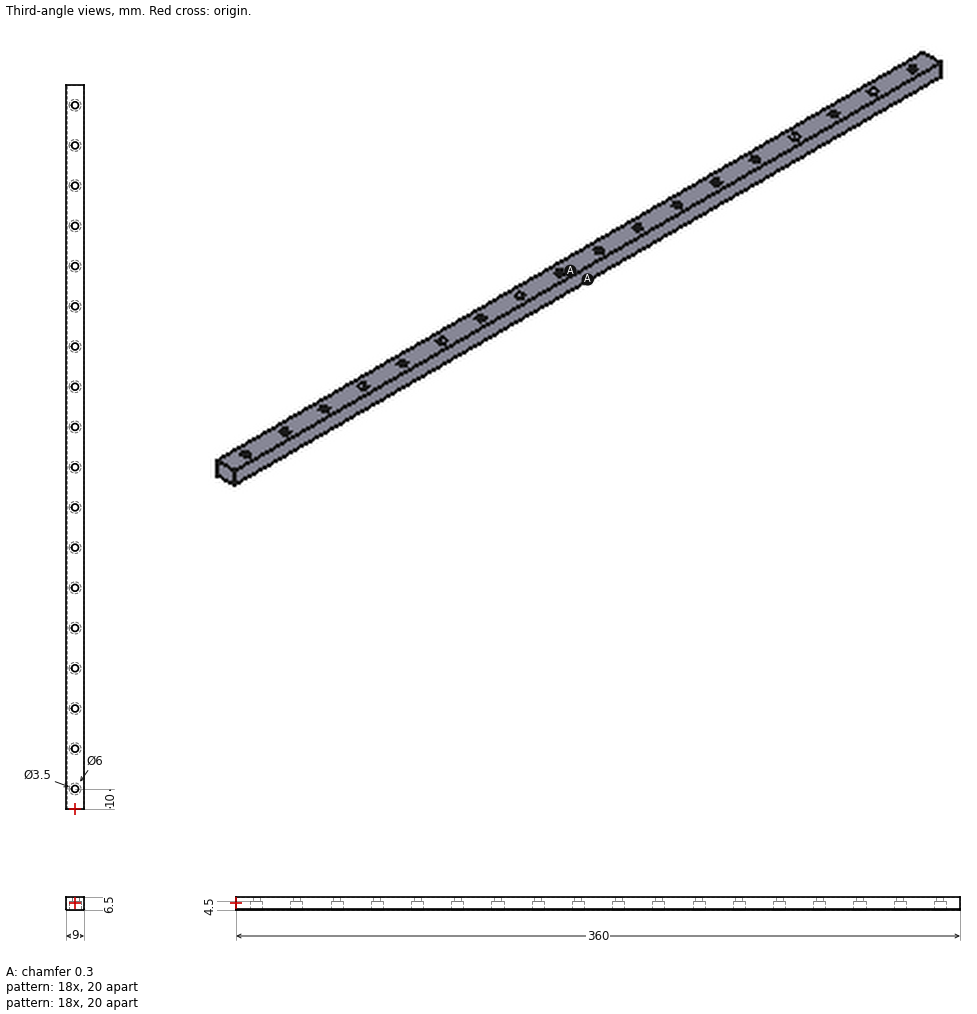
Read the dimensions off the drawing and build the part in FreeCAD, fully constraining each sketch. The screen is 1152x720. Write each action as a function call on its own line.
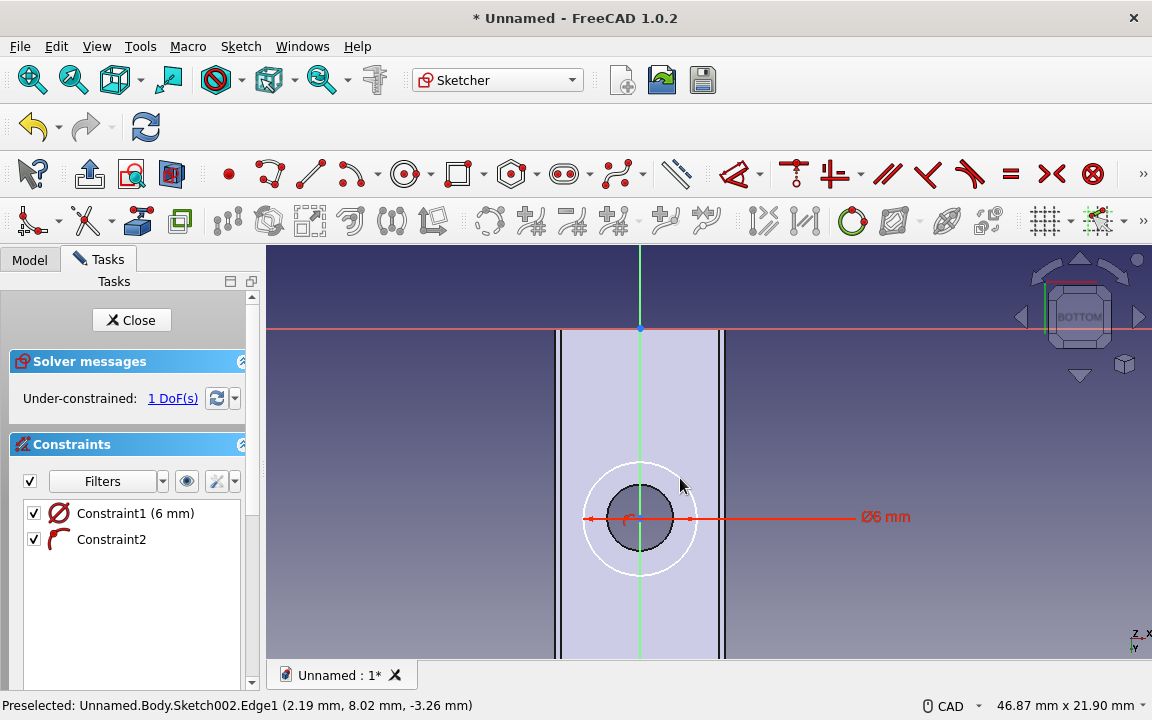
key(d)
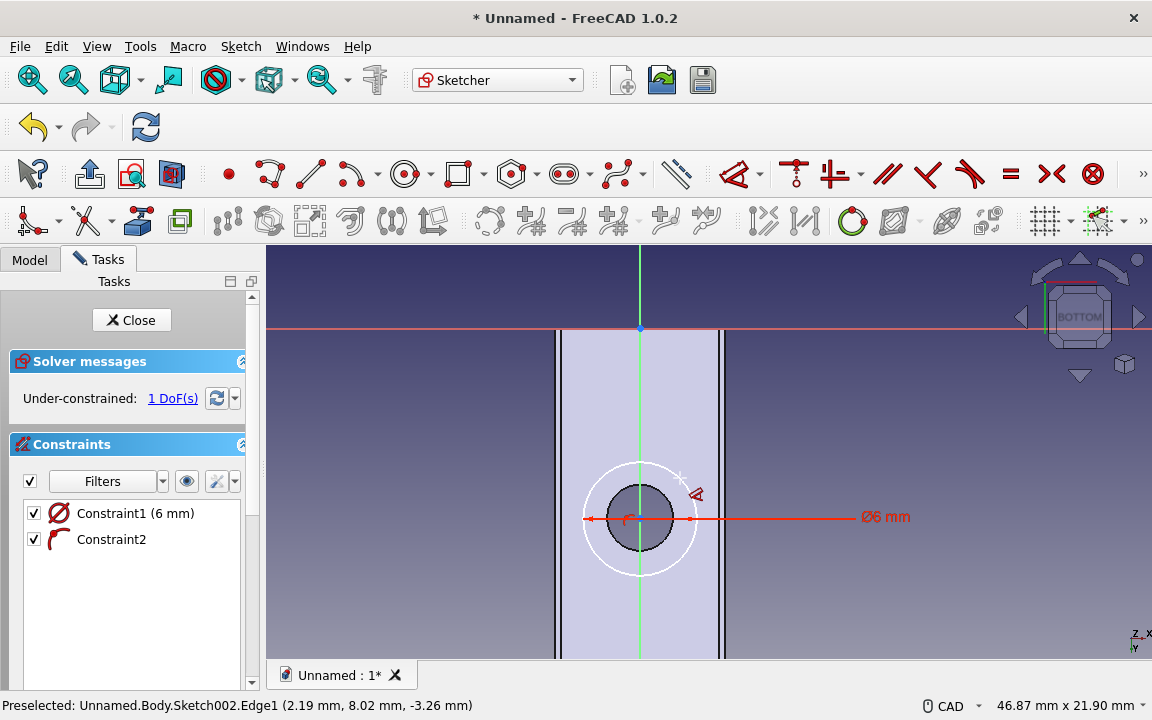
click(640, 519)
click(674, 424)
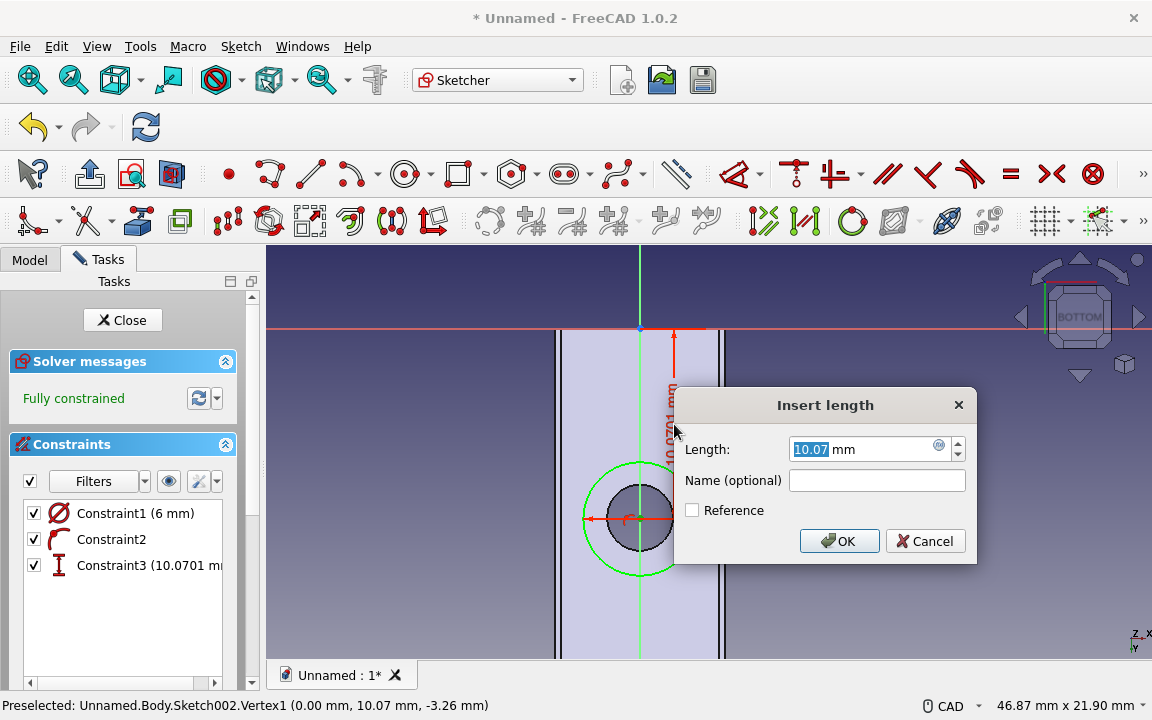
text(10)
key(Return)
key(Escape)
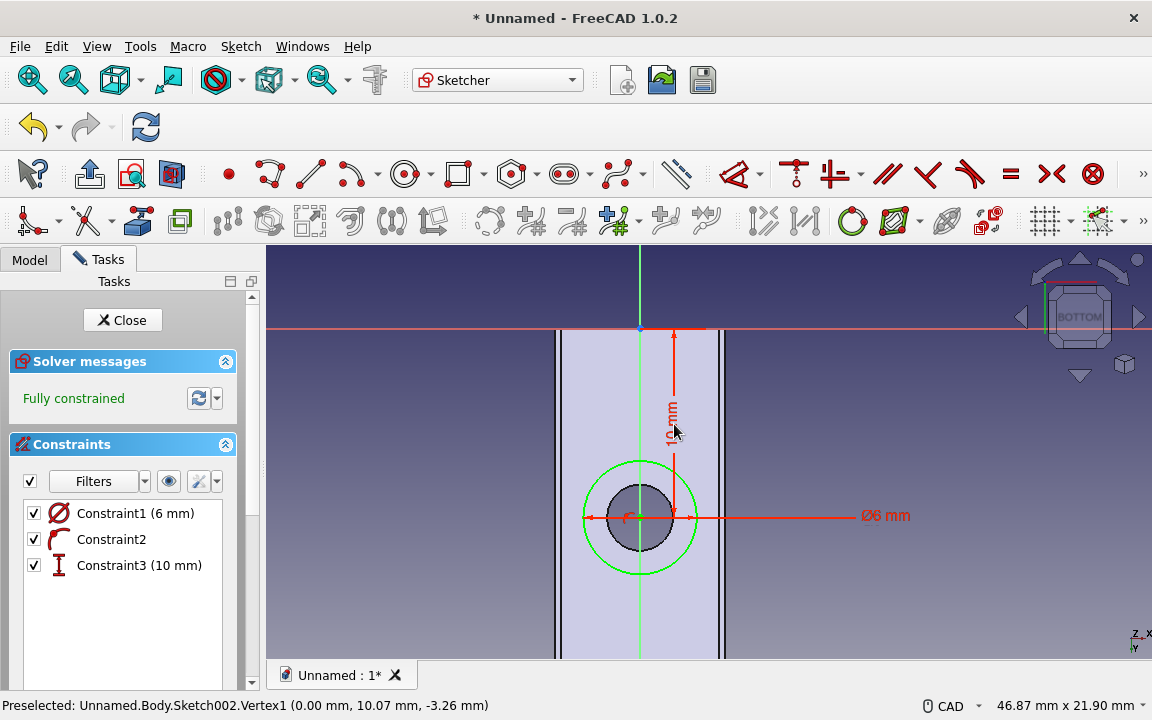
click(123, 320)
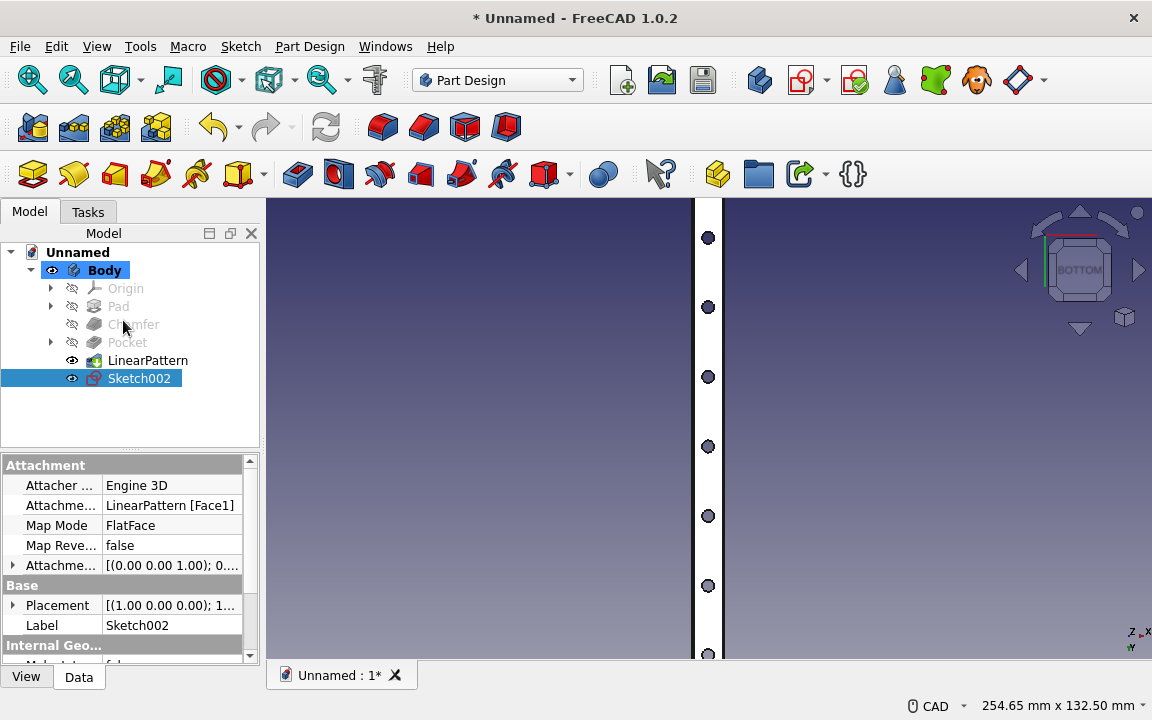
click(298, 174)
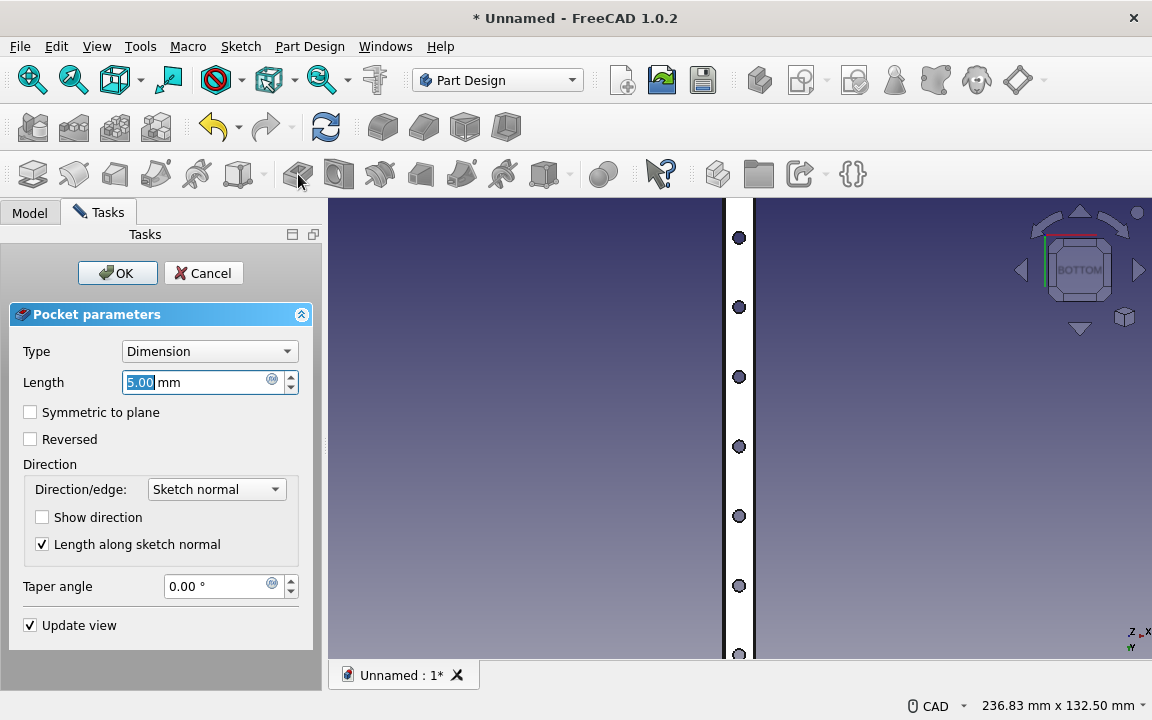
text(4.5)
key(Tab)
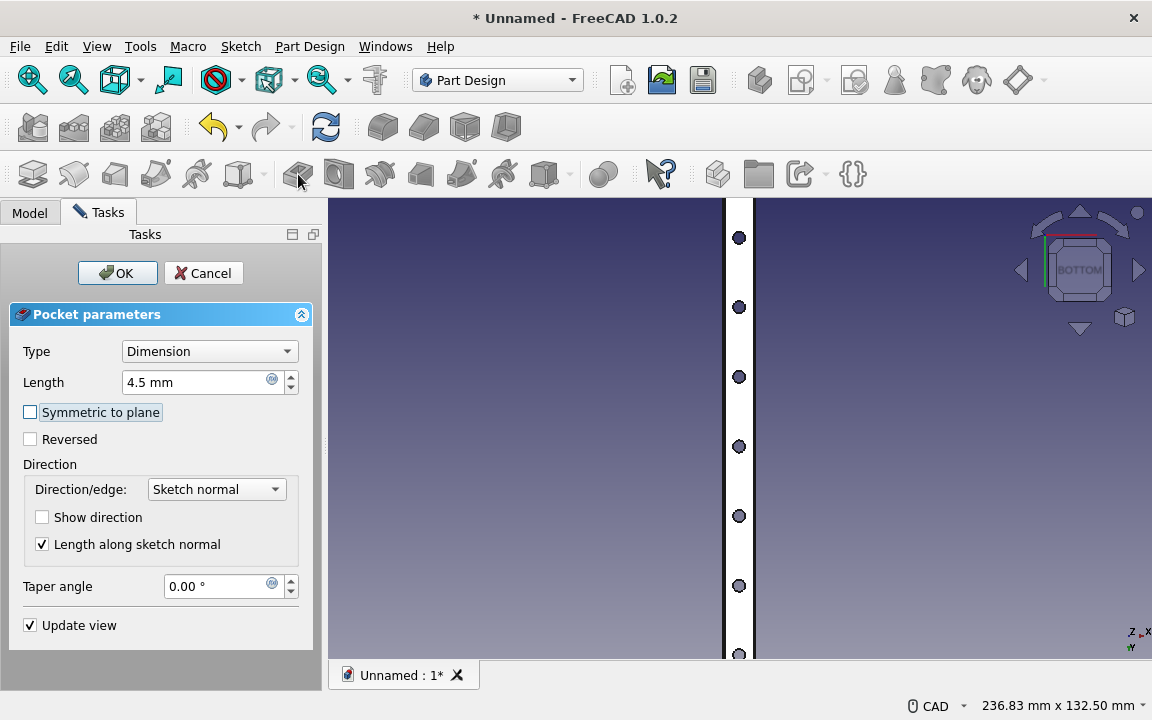
click(118, 273)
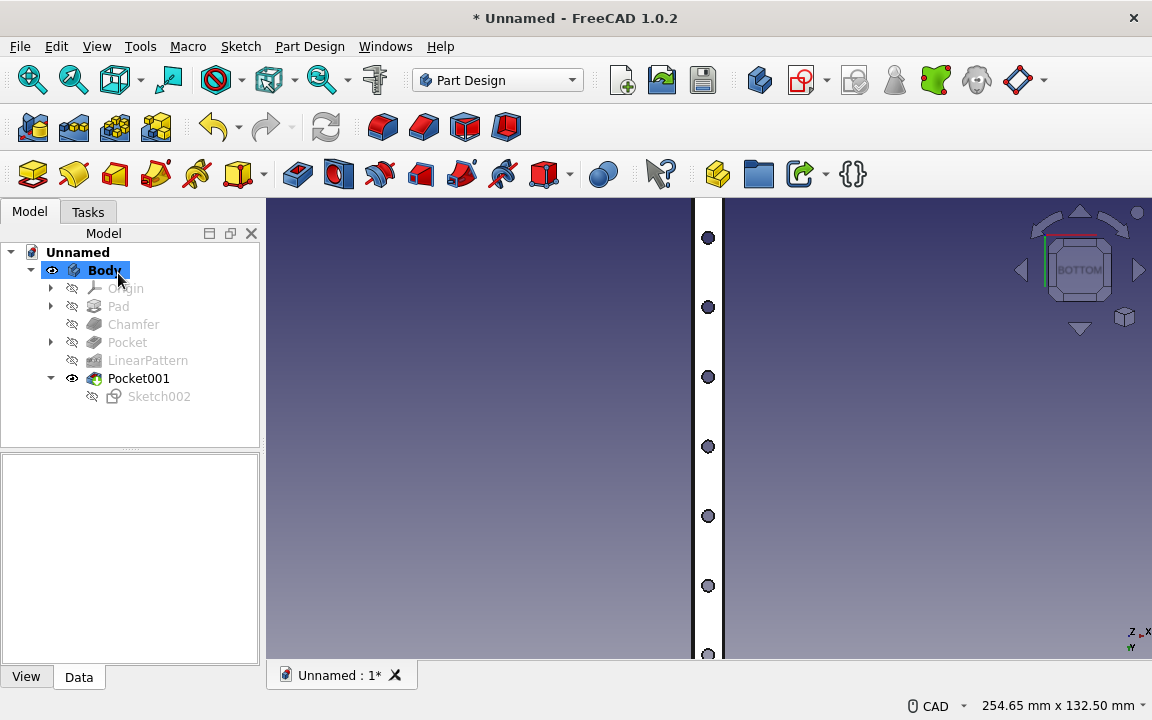
key(v)
key(f)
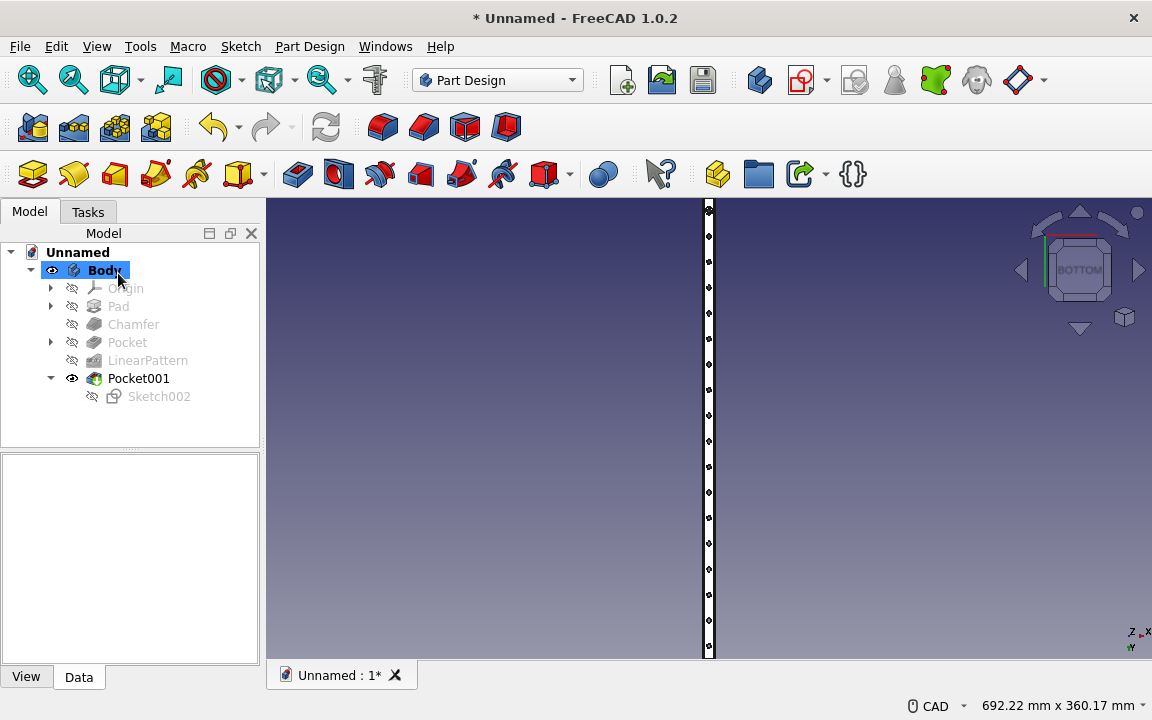
click(117, 378)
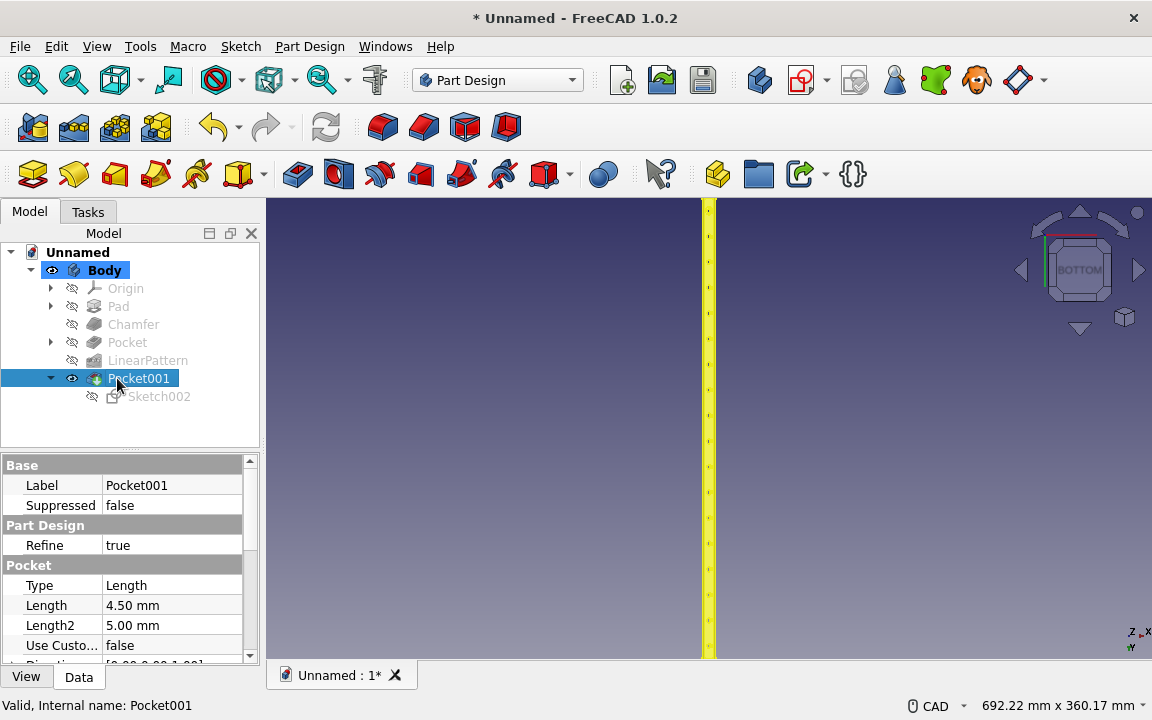
click(74, 128)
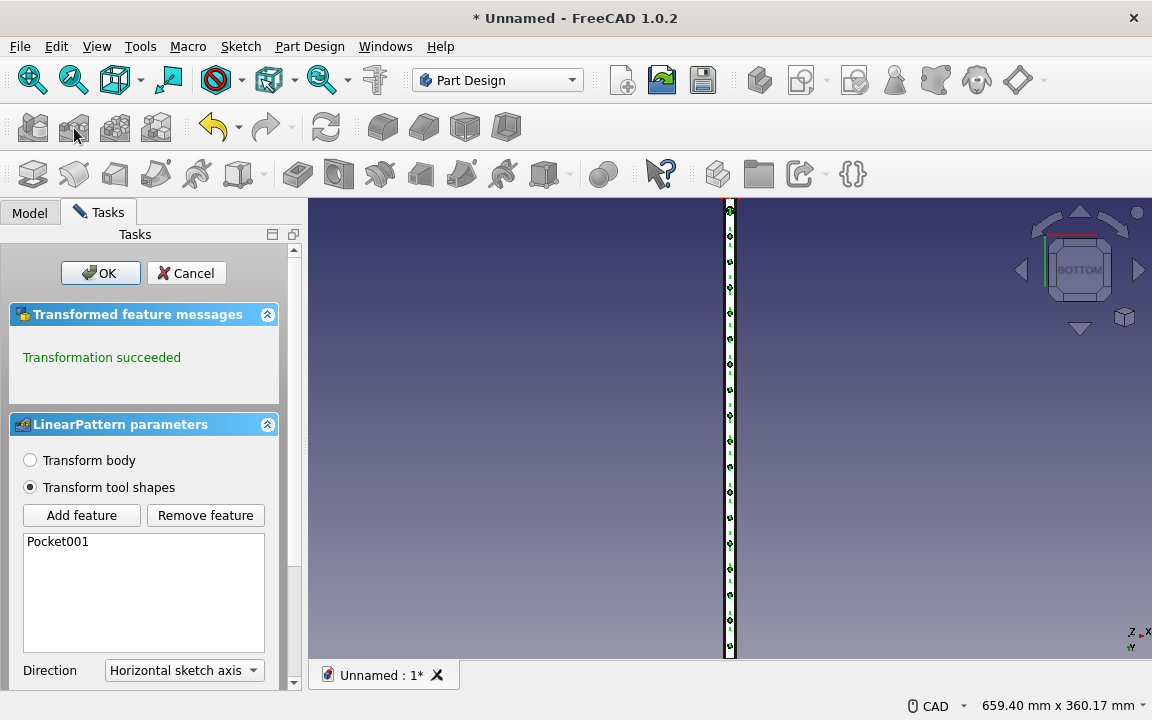
click(185, 670)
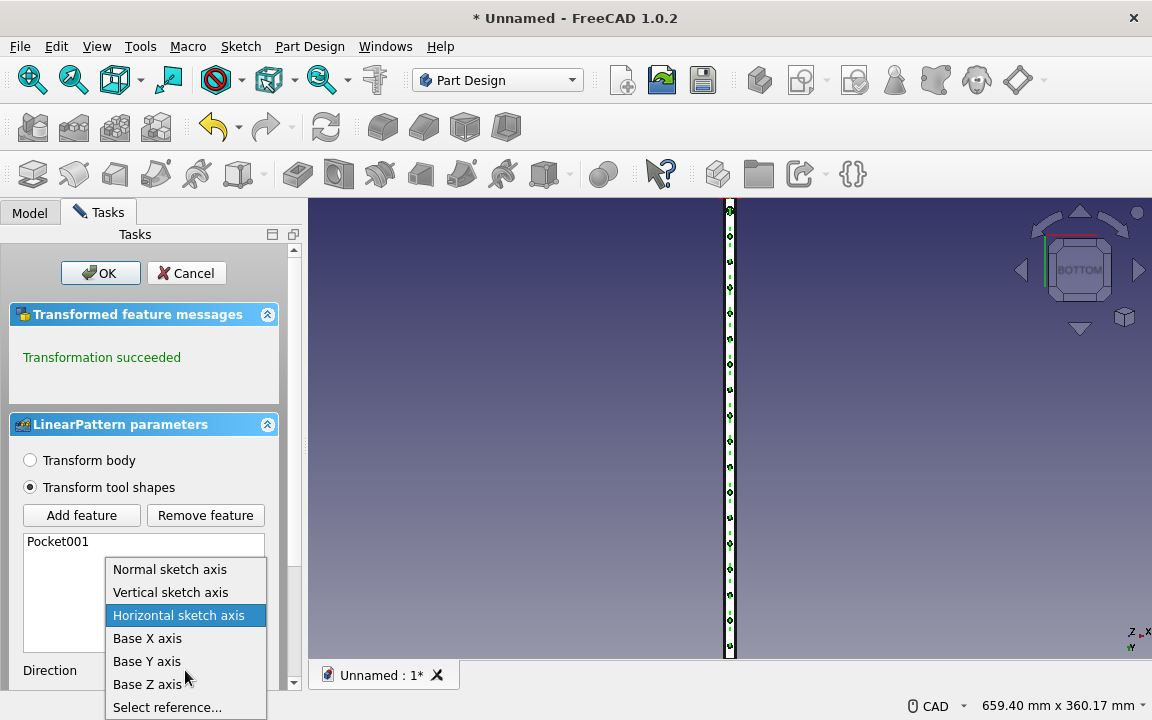
click(184, 662)